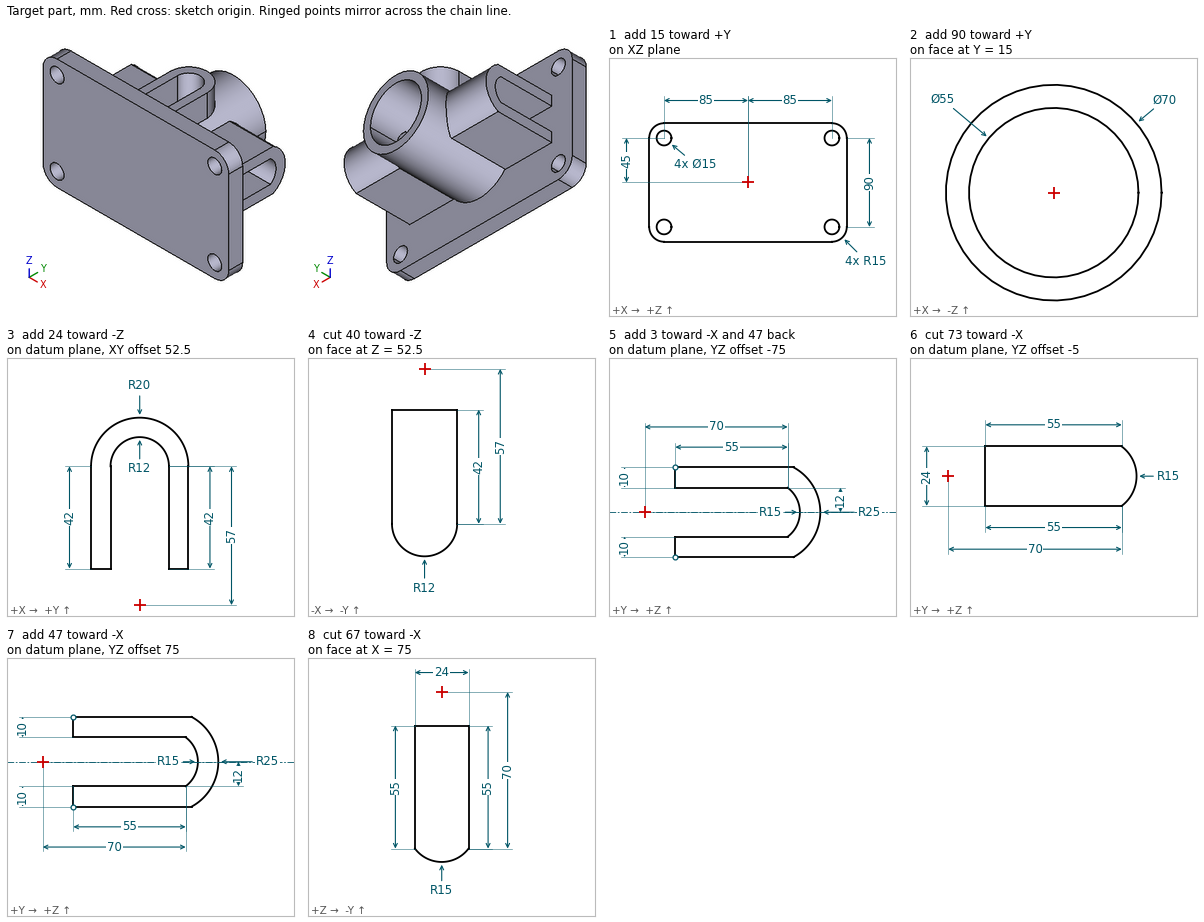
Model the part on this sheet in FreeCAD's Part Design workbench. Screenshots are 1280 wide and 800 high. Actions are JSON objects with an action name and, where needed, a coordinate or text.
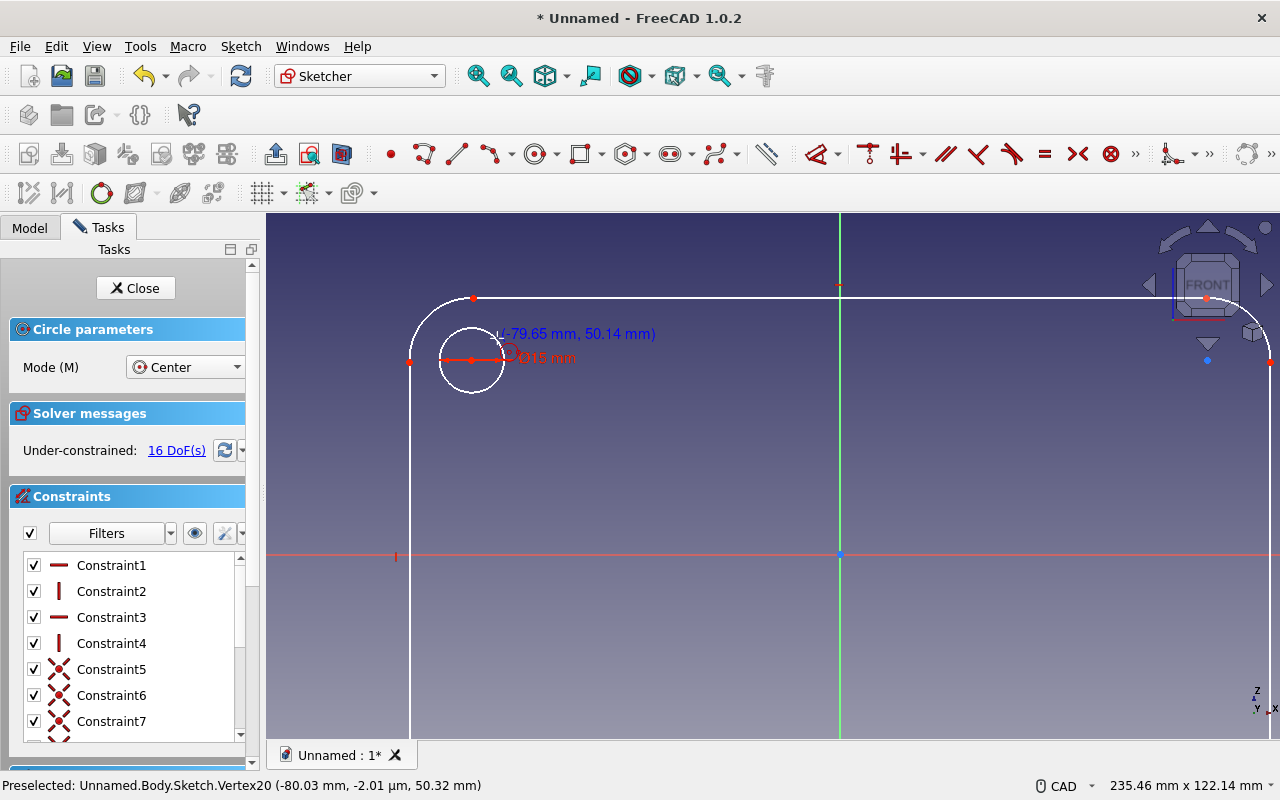
{"action": "scroll", "coordinate": [429, 316], "scroll_direction": "down", "scroll_amount": 2}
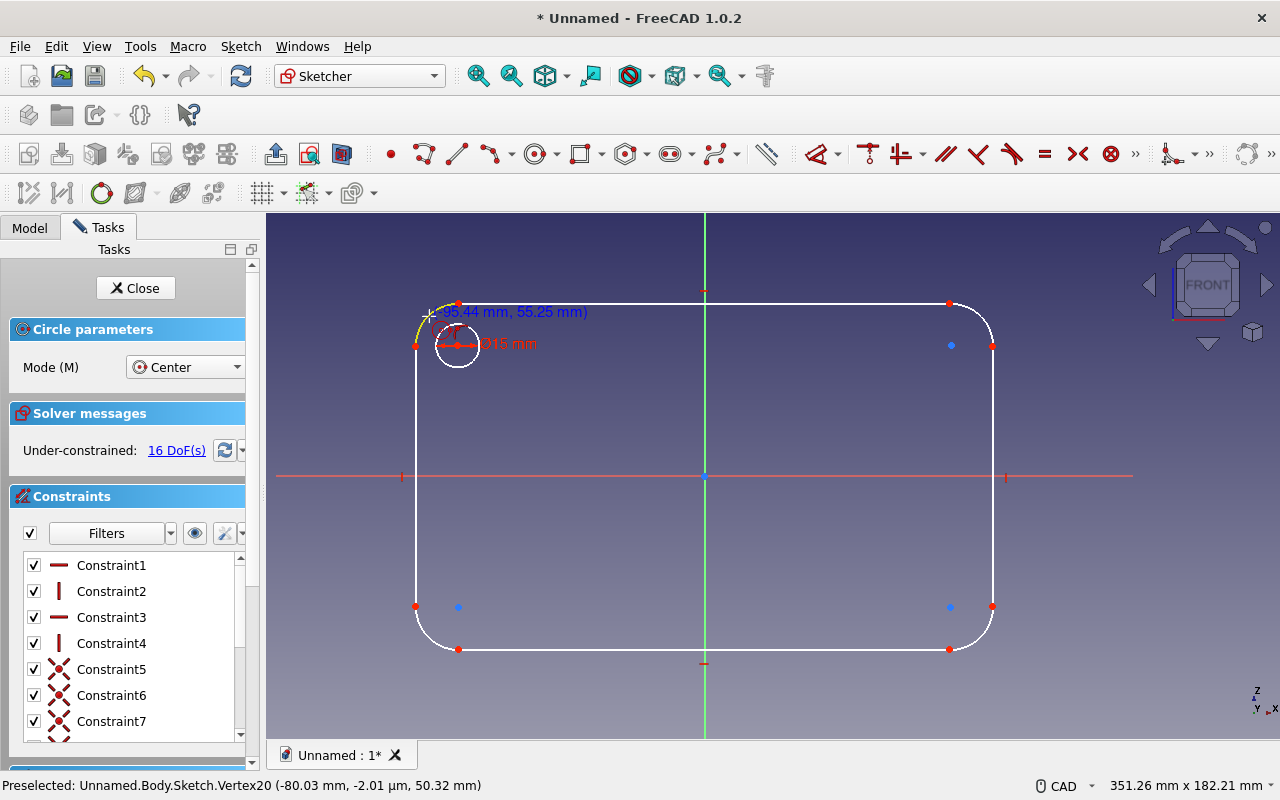
{"action": "left_click", "coordinate": [950, 346]}
{"action": "mouse_move", "coordinate": [965, 331]}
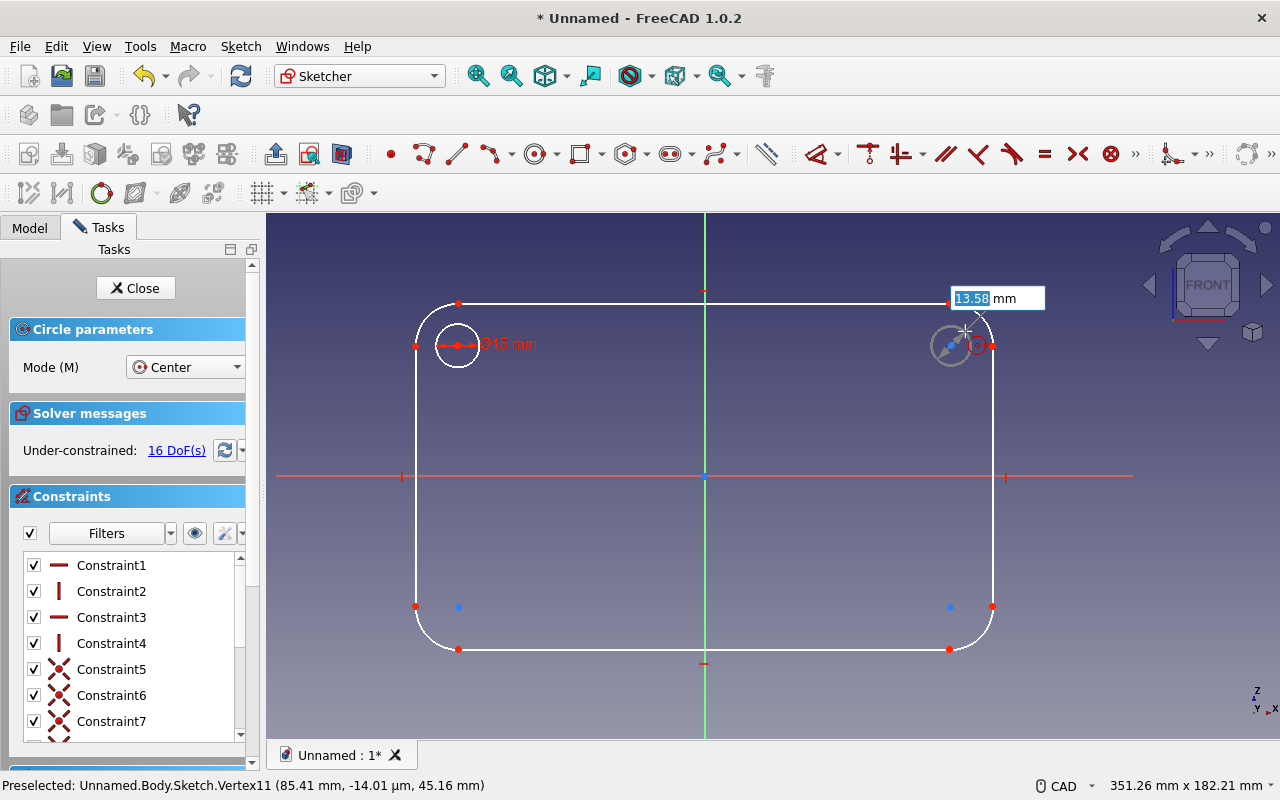
{"action": "type", "text": "15"}
{"action": "key", "text": "Return"}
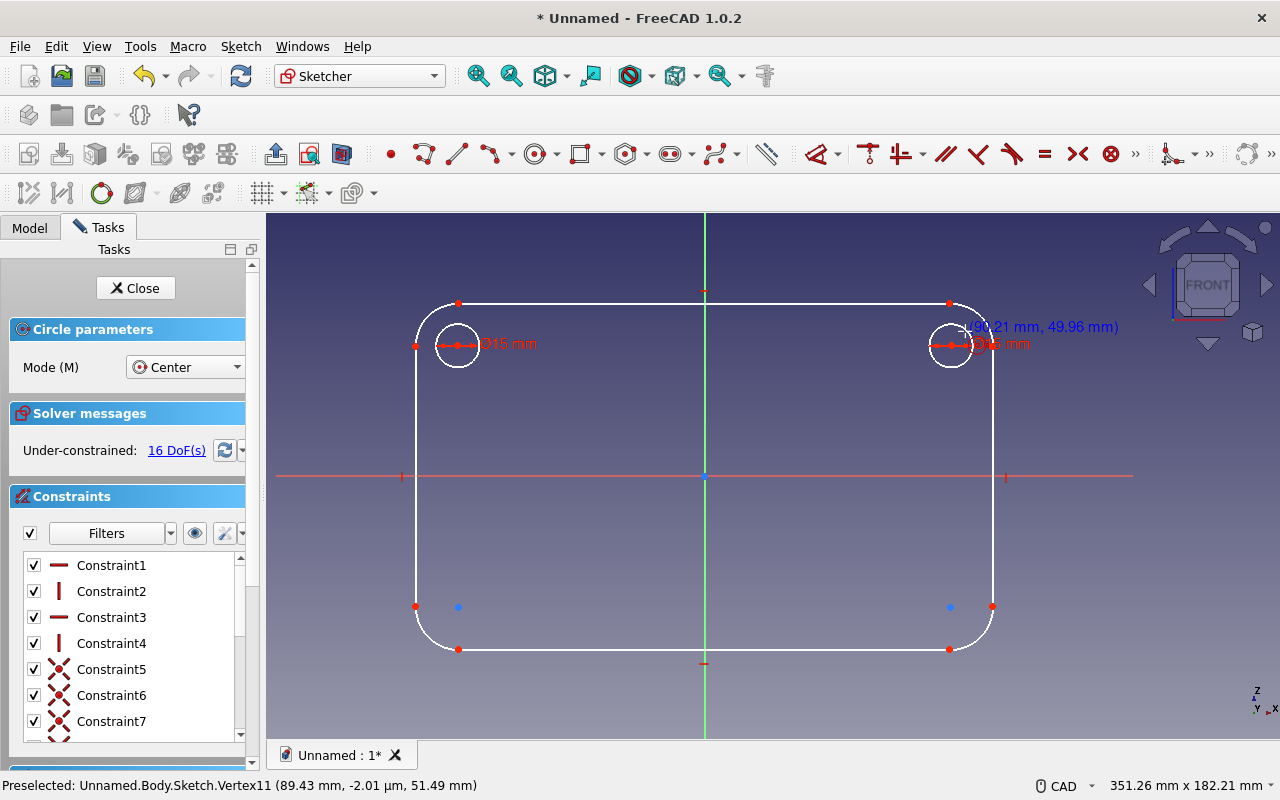
{"action": "left_click", "coordinate": [459, 606]}
{"action": "mouse_move", "coordinate": [475, 591]}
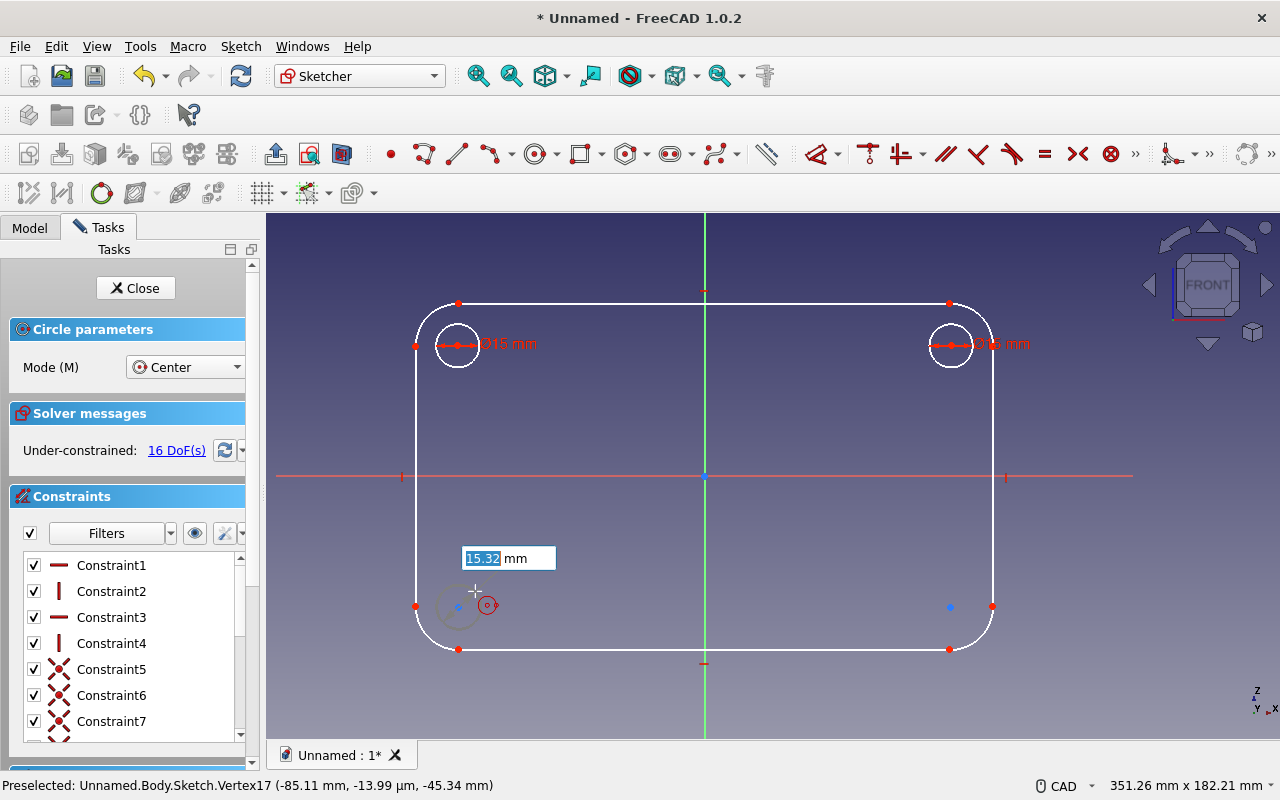
{"action": "type", "text": "15"}
{"action": "key", "text": "Return"}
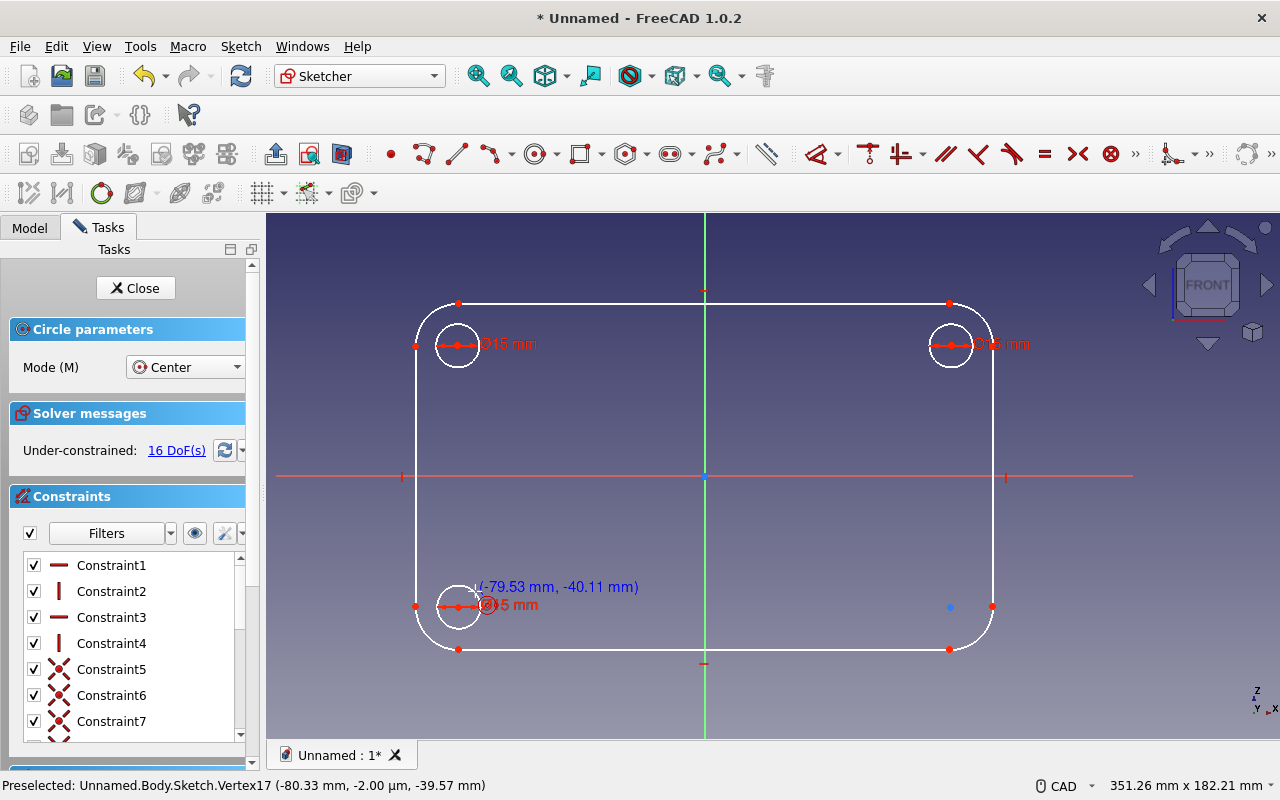
{"action": "left_click", "coordinate": [950, 606]}
{"action": "mouse_move", "coordinate": [965, 591]}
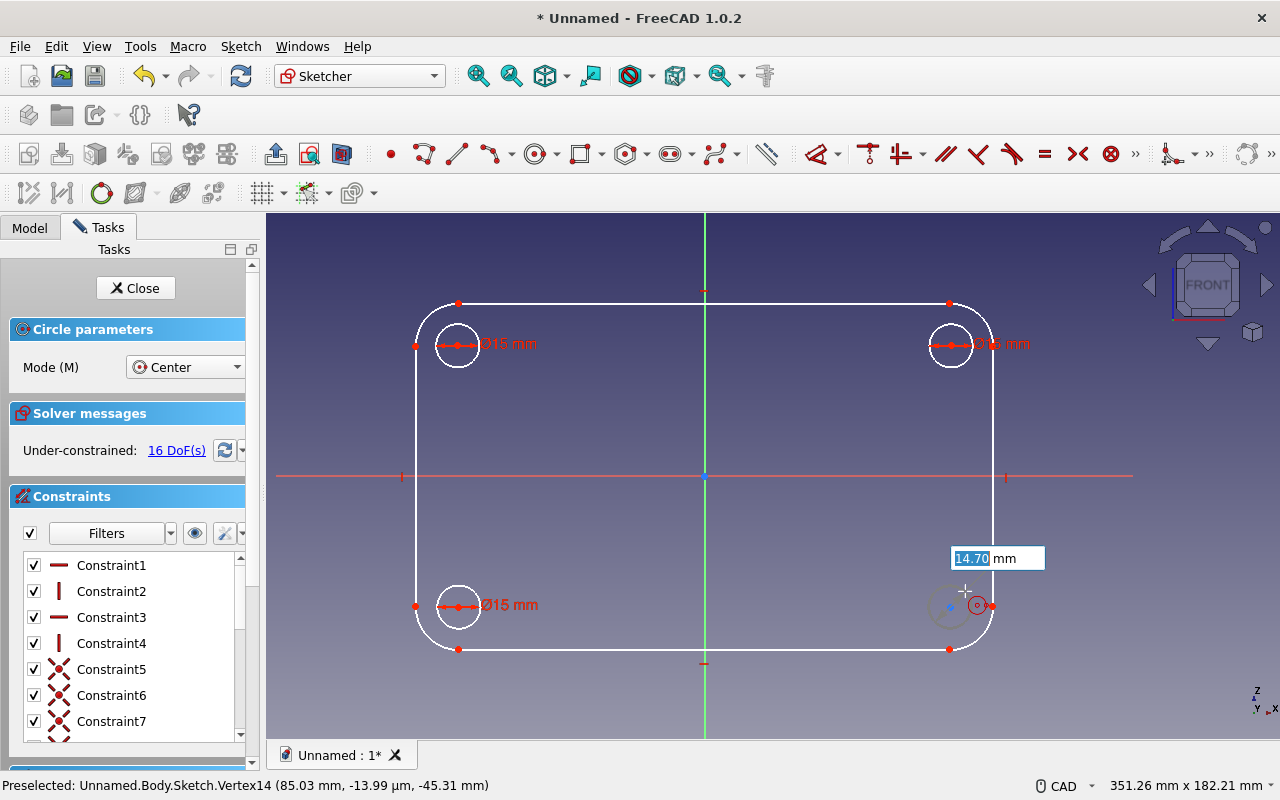
{"action": "type", "text": "15"}
{"action": "key", "text": "Return"}
{"action": "key", "text": "Escape"}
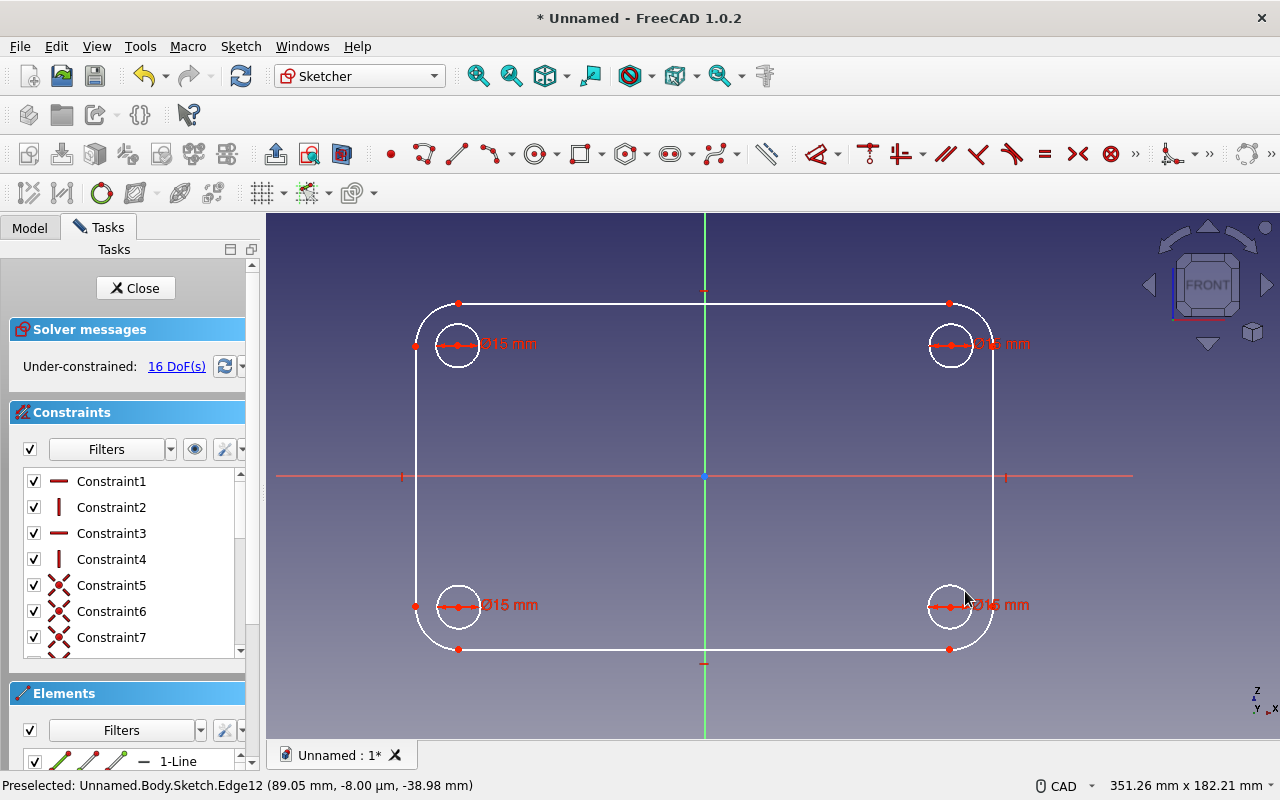
{"action": "left_click", "coordinate": [606, 304]}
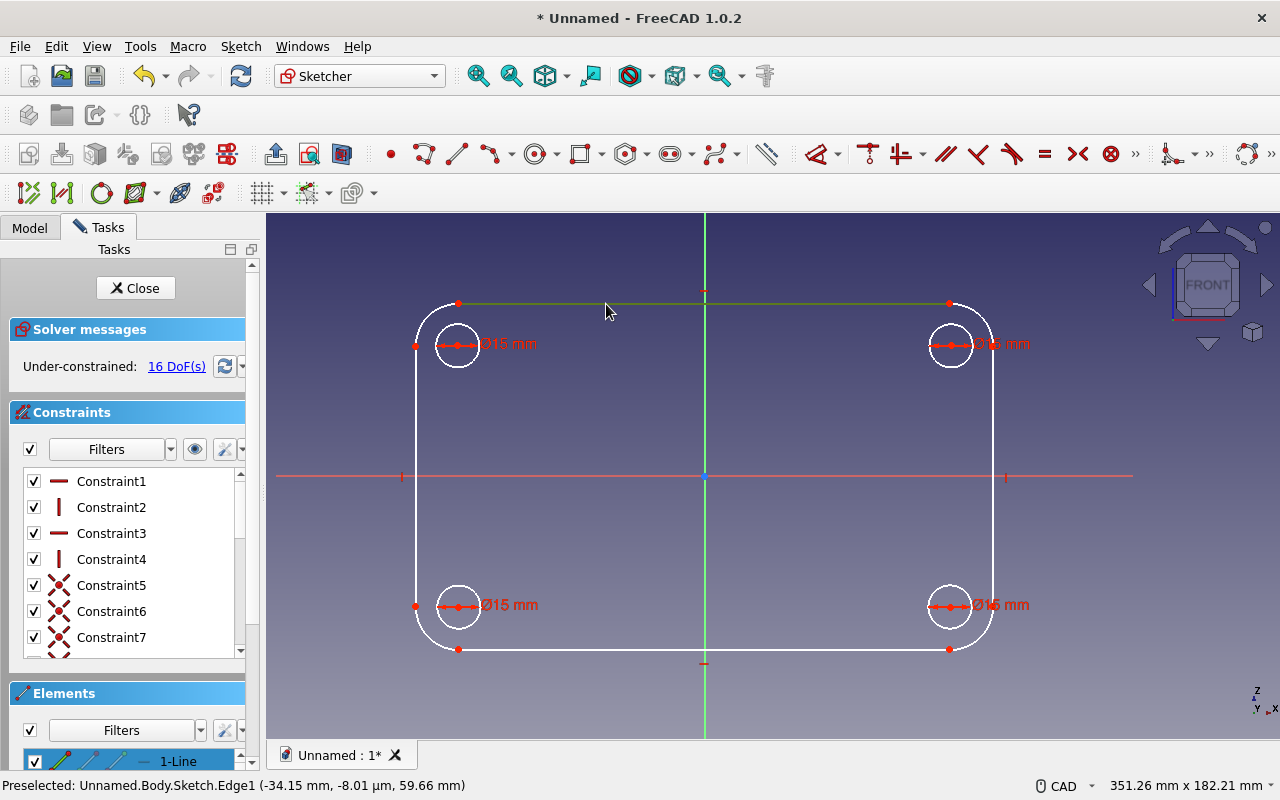
{"action": "left_click", "coordinate": [989, 327]}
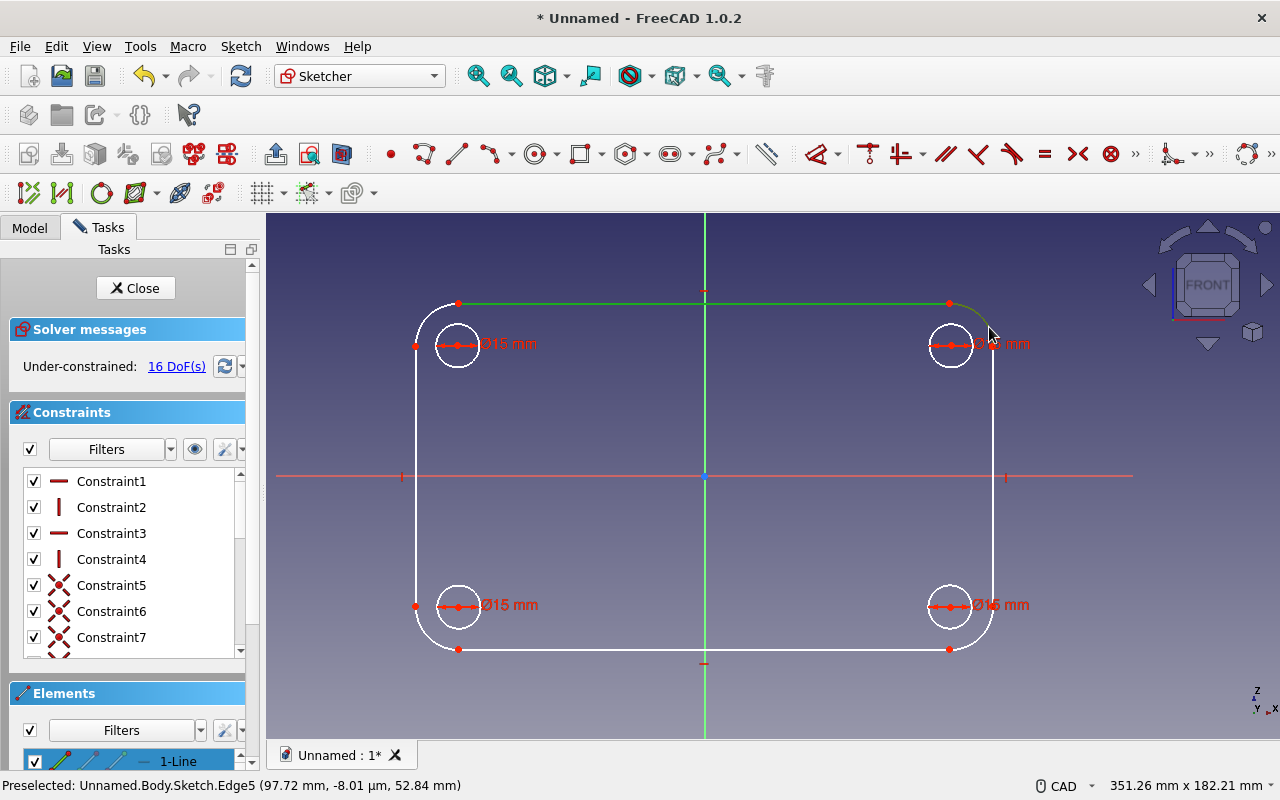
{"action": "left_click", "coordinate": [1012, 154]}